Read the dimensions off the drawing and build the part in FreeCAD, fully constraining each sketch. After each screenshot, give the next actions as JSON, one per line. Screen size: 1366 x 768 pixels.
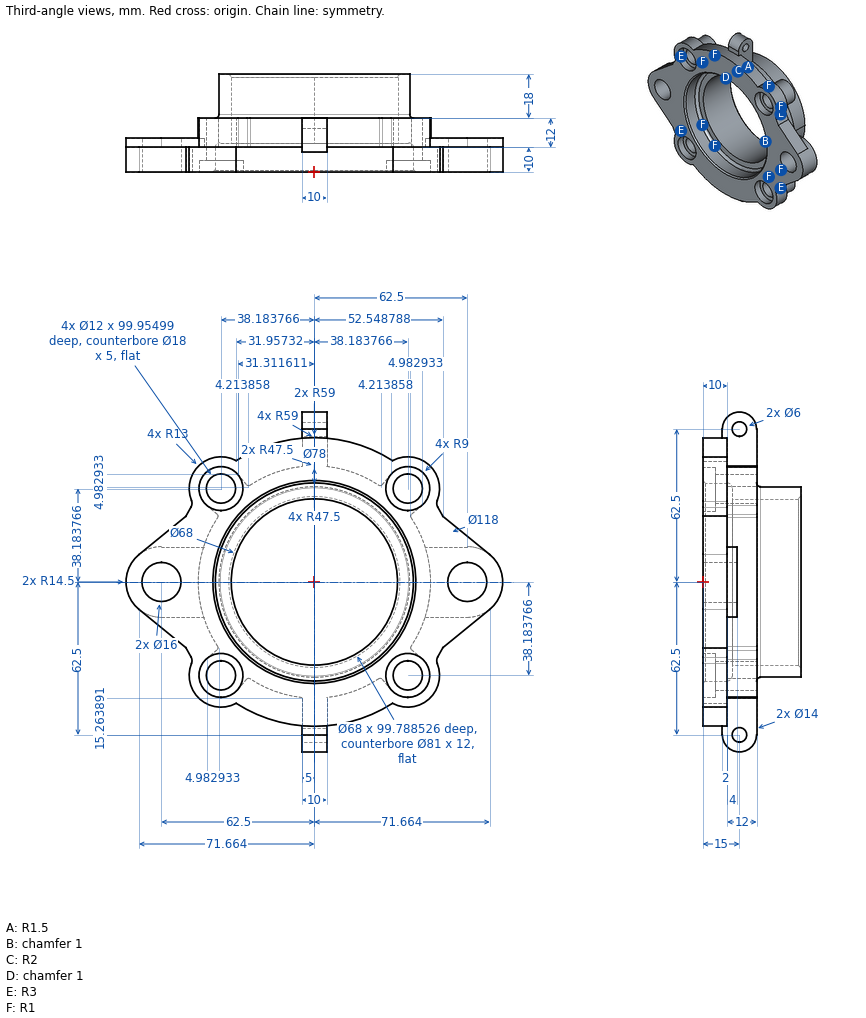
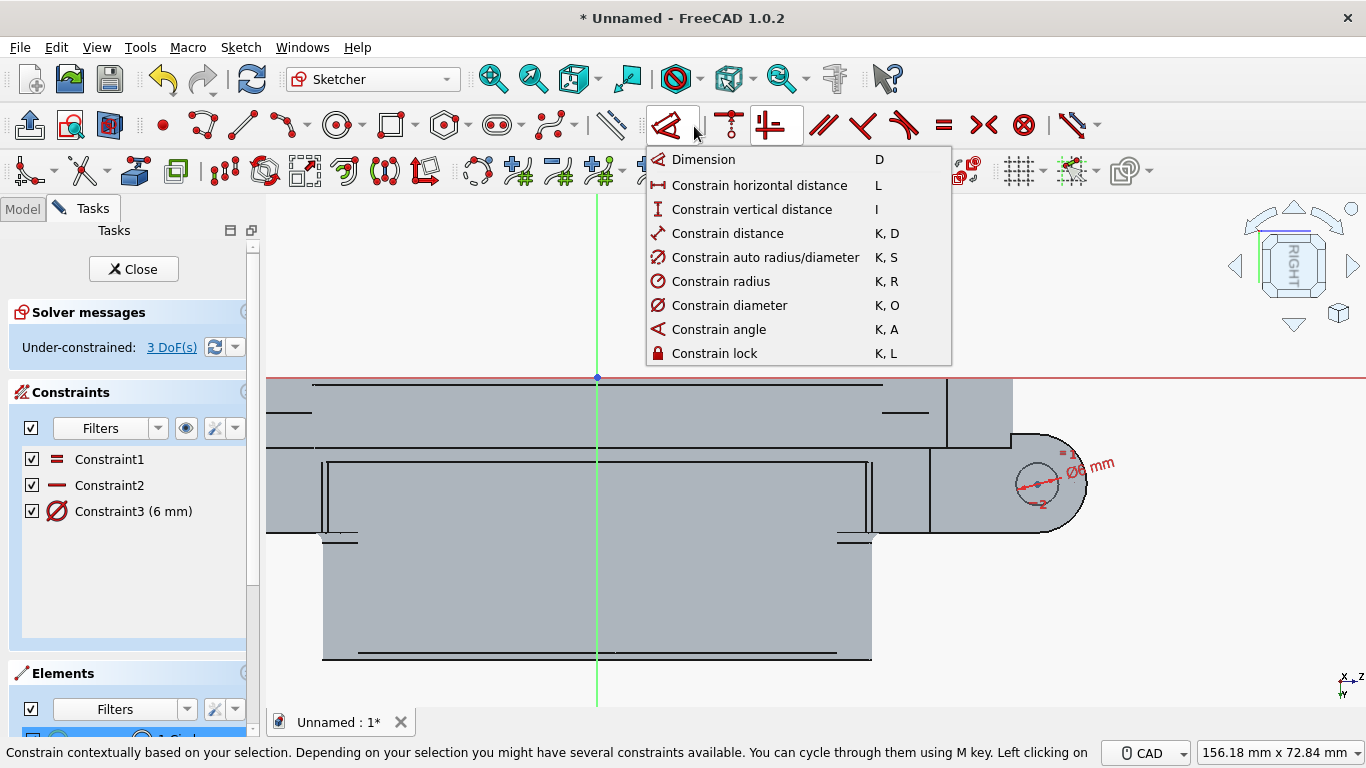
{"action": "left_click", "coordinate": [799, 209]}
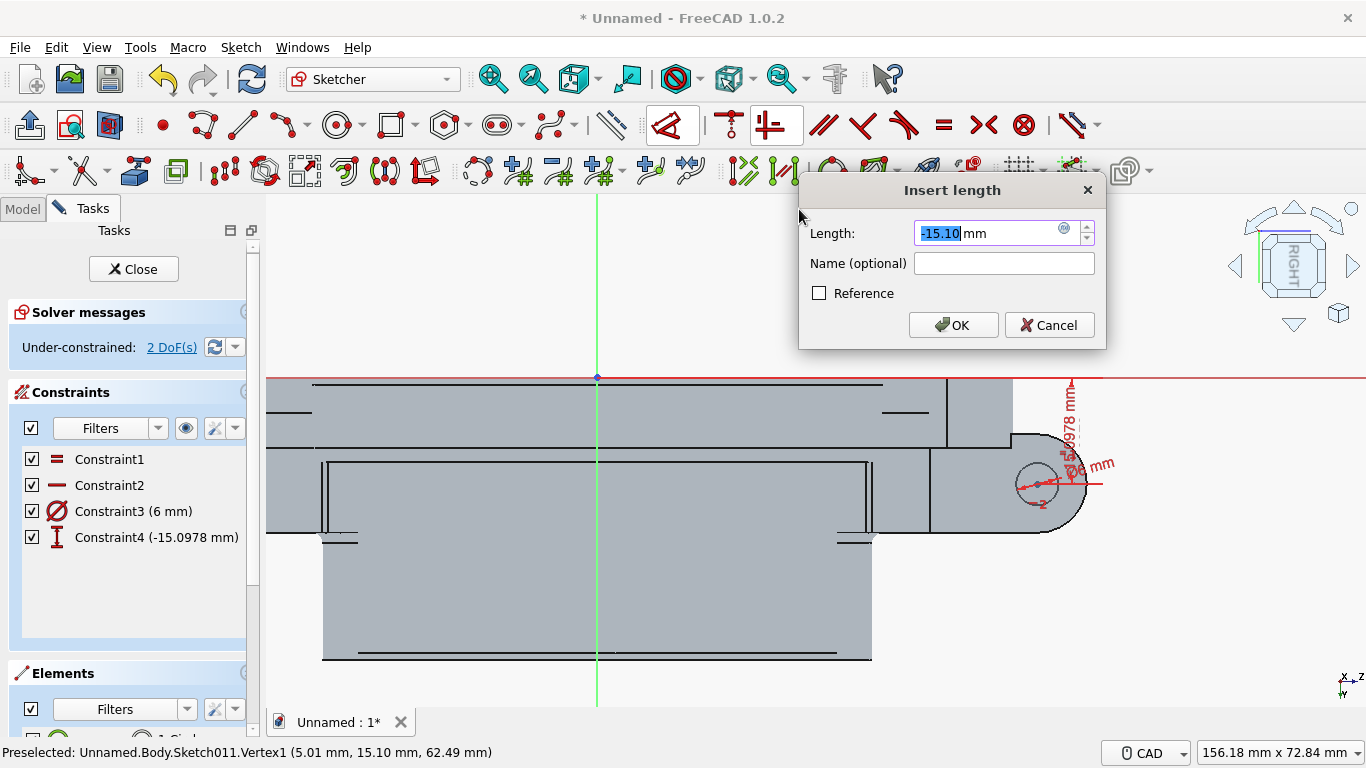
{"action": "type", "text": "-15"}
{"action": "key", "text": "Return"}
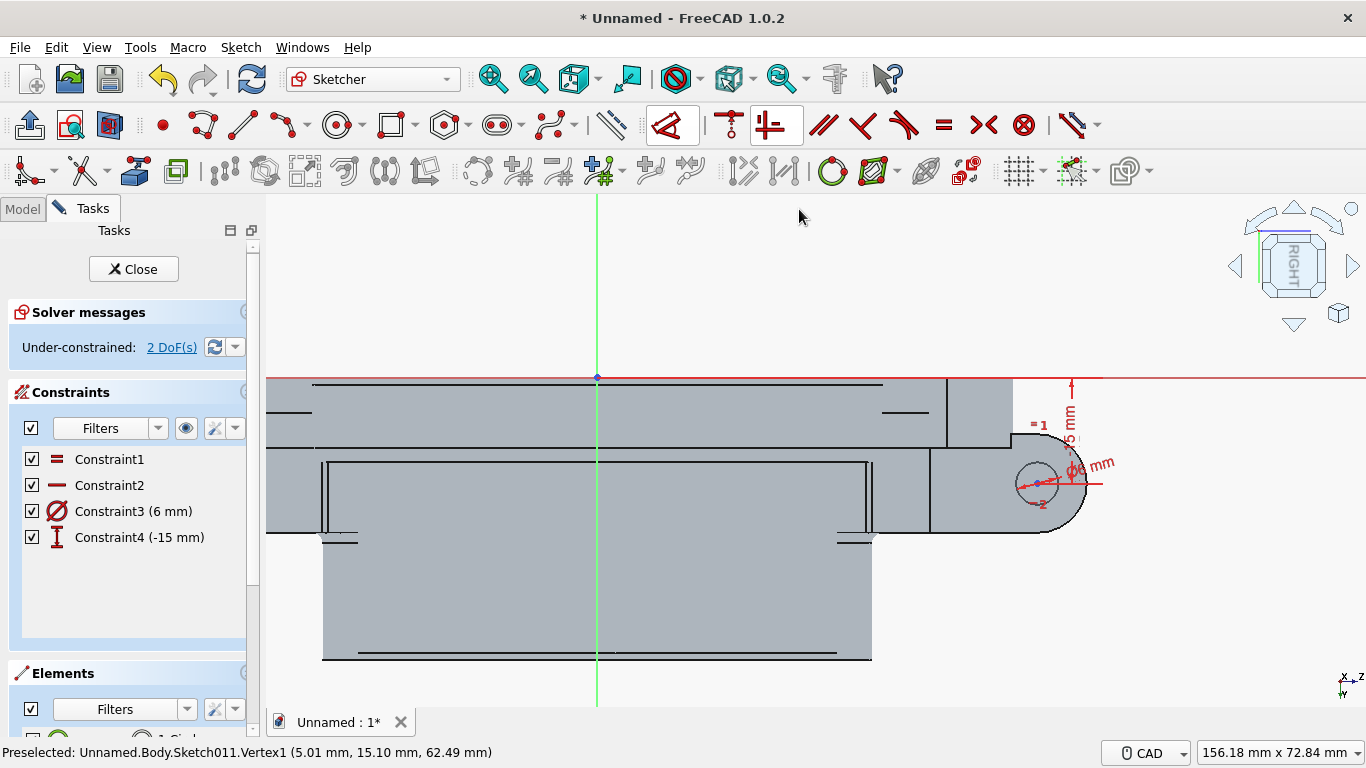
{"action": "left_click", "coordinate": [1037, 484]}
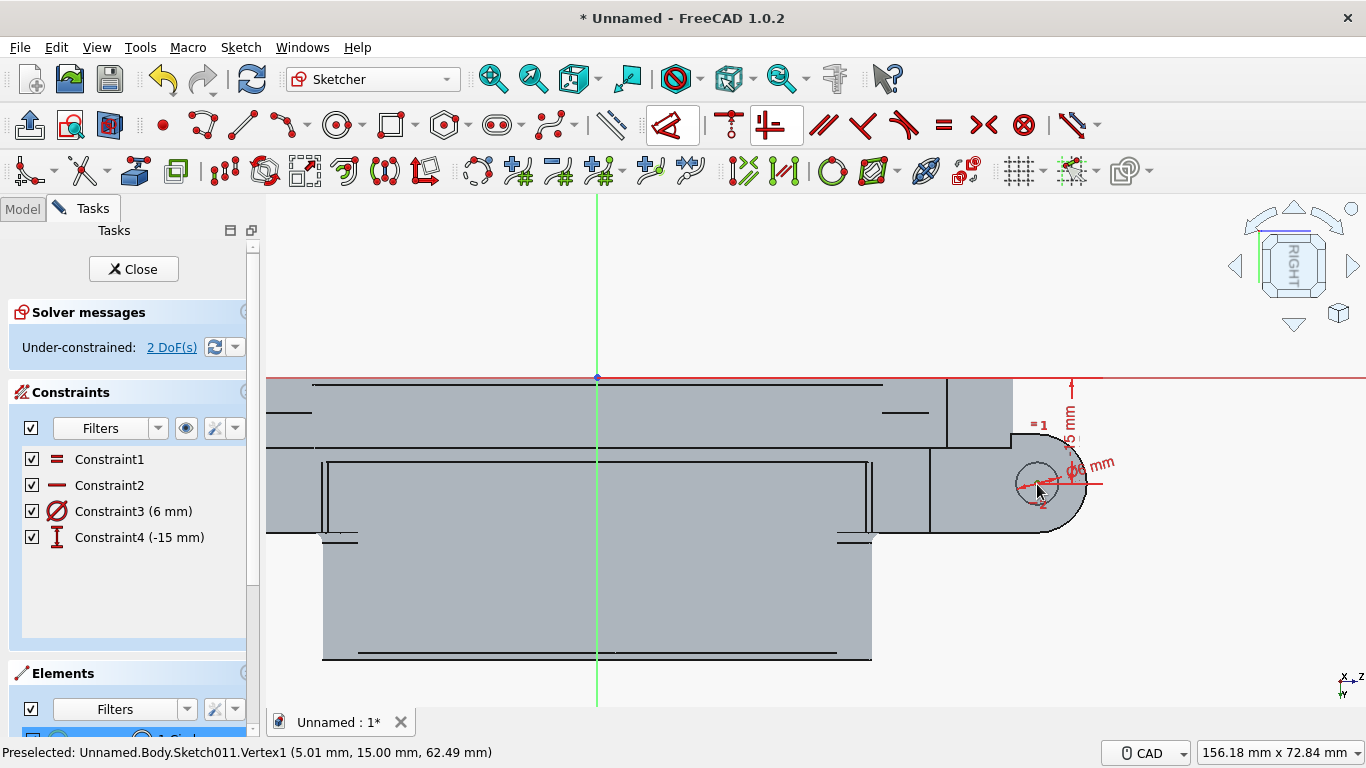
{"action": "left_click", "coordinate": [694, 126]}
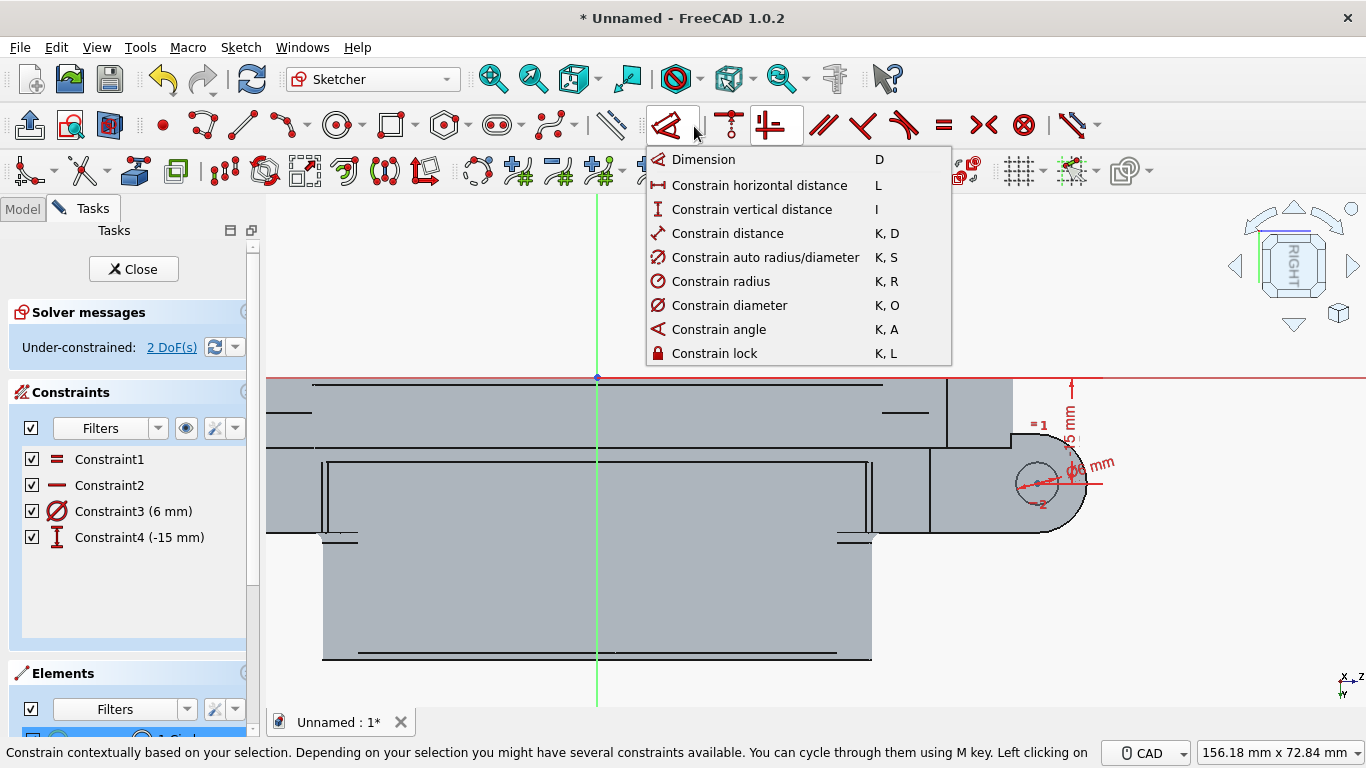
{"action": "left_click", "coordinate": [799, 185]}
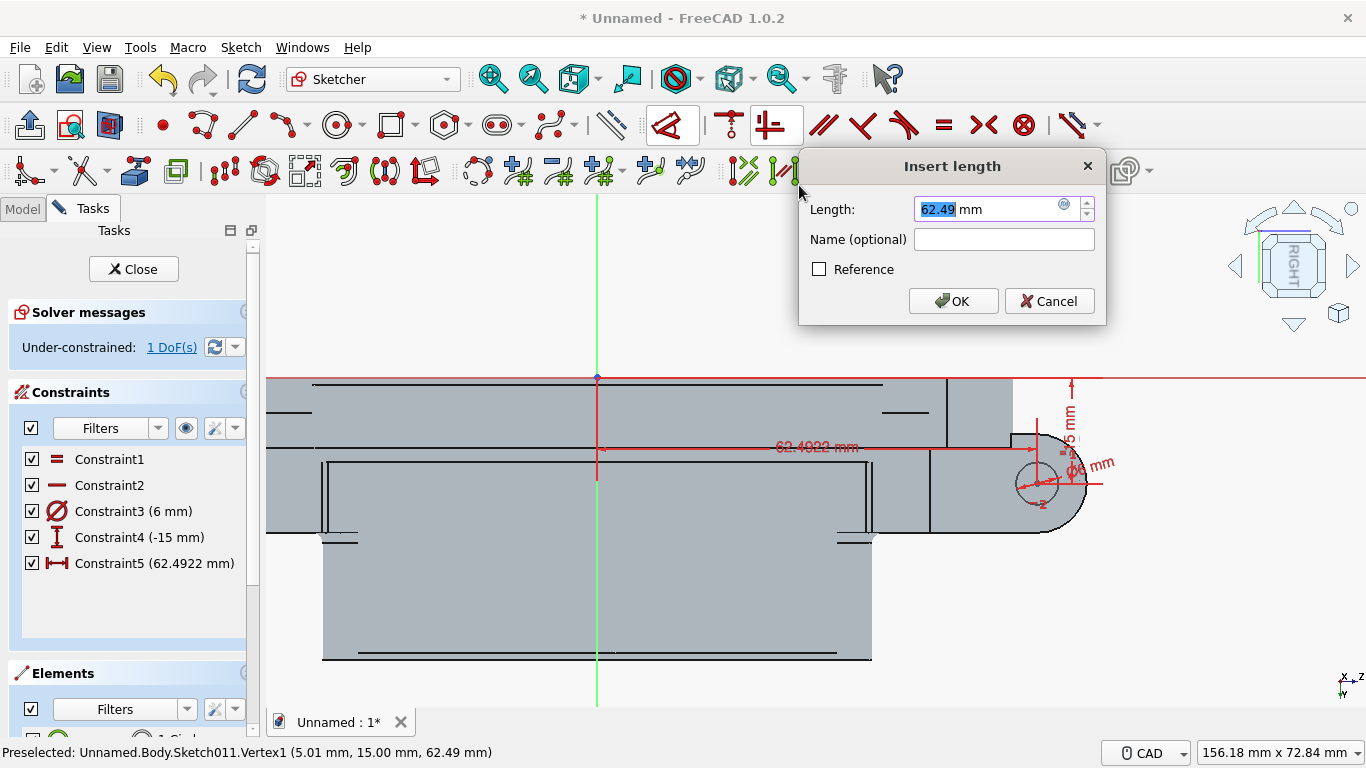
{"action": "type", "text": "62.5"}
{"action": "key", "text": "Return"}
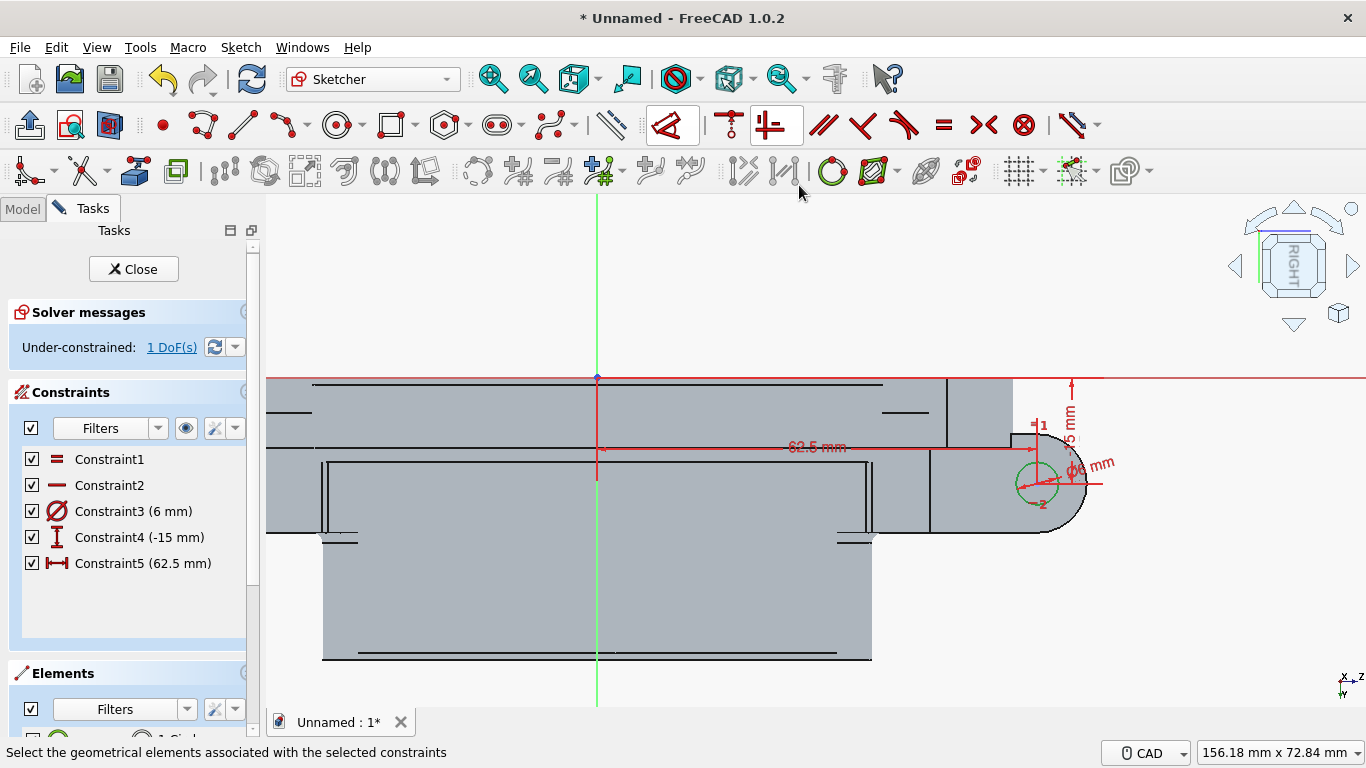
{"action": "scroll", "coordinate": [1053, 469], "scroll_direction": "down", "scroll_amount": 2}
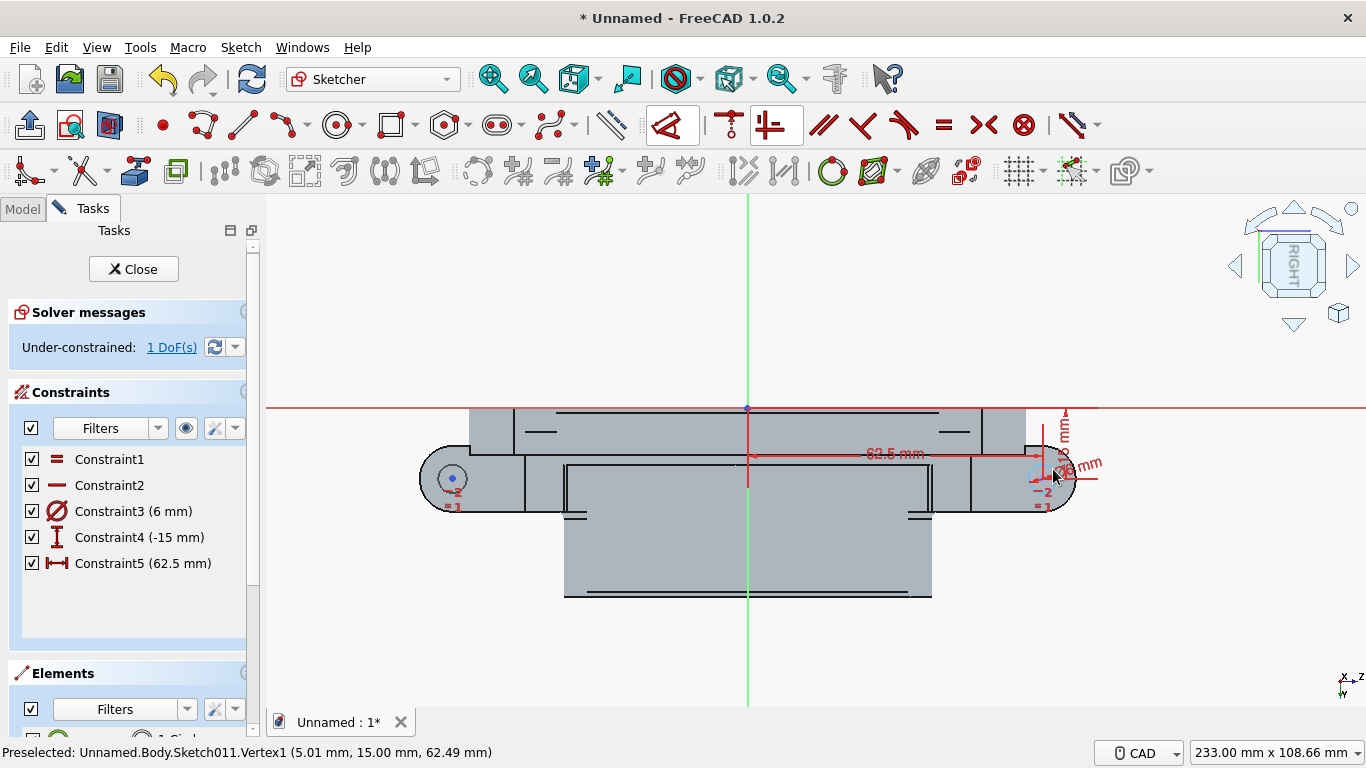
{"action": "left_click", "coordinate": [453, 479]}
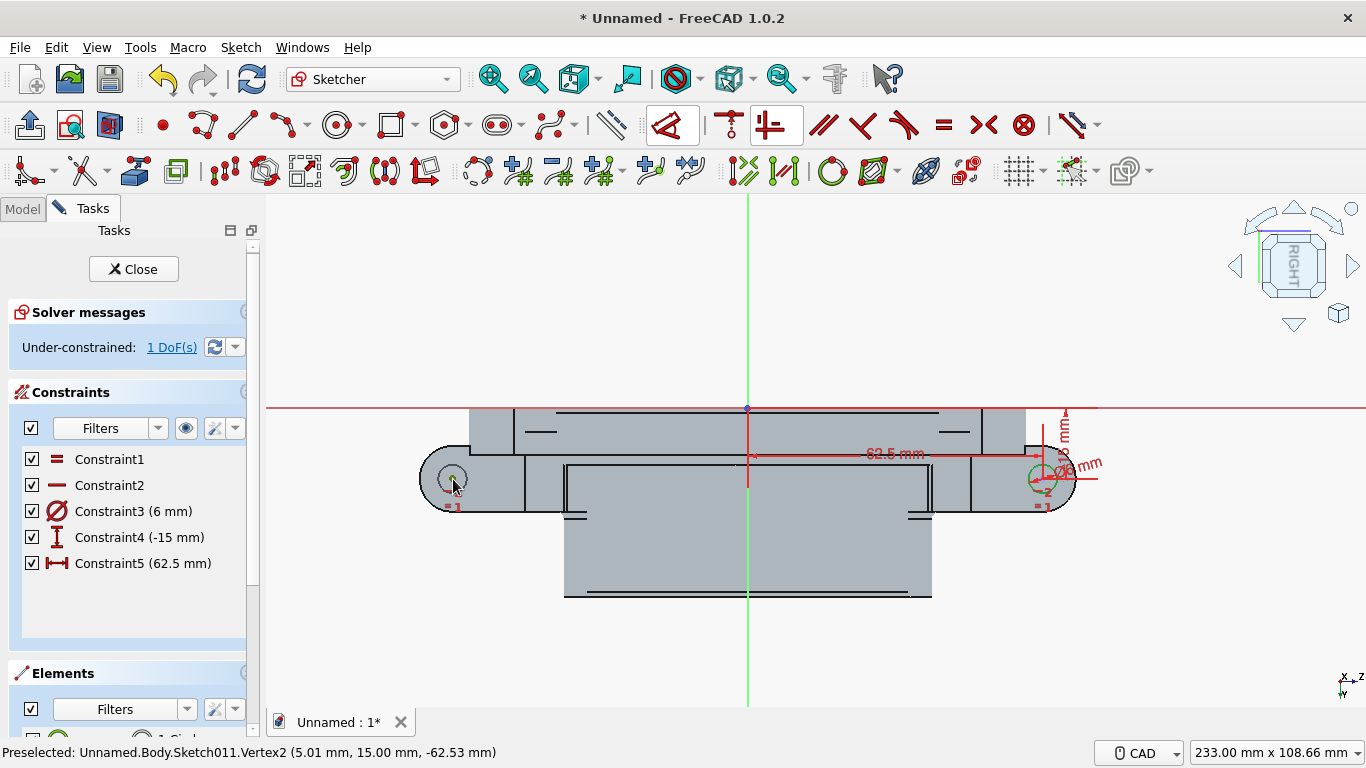
{"action": "left_click", "coordinate": [694, 126]}